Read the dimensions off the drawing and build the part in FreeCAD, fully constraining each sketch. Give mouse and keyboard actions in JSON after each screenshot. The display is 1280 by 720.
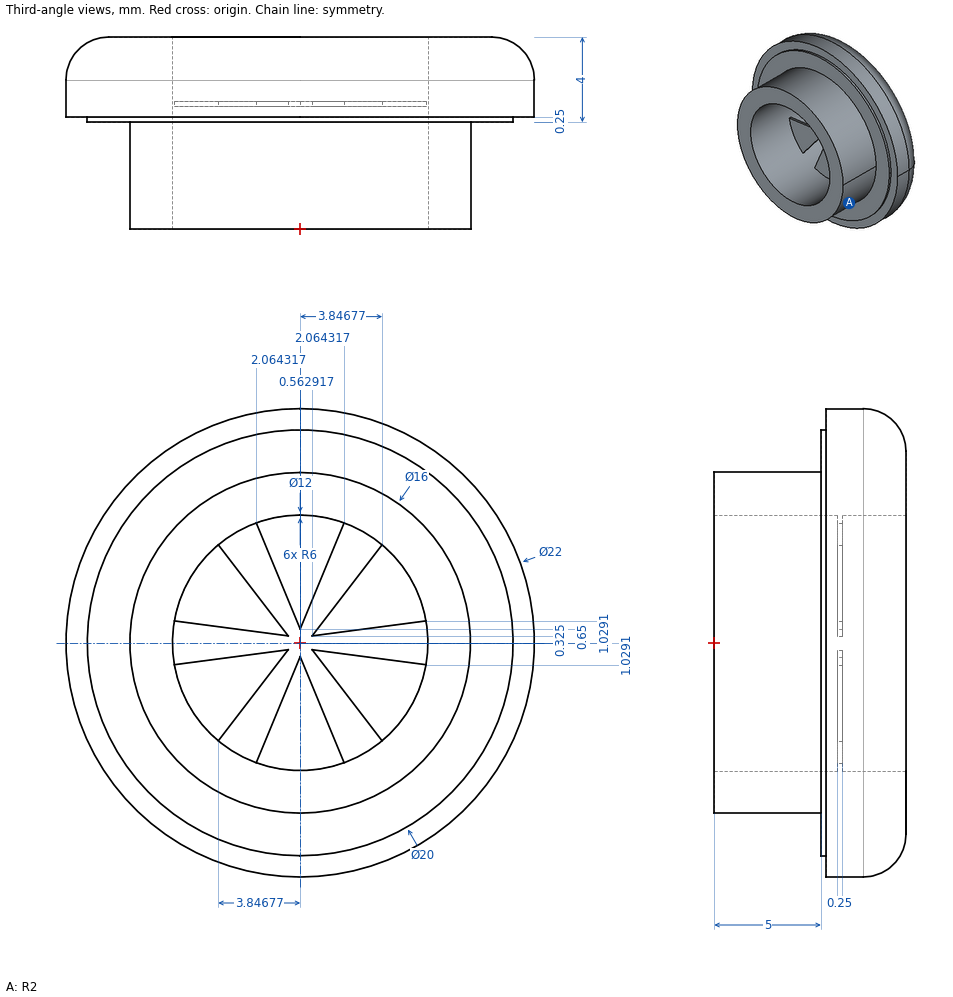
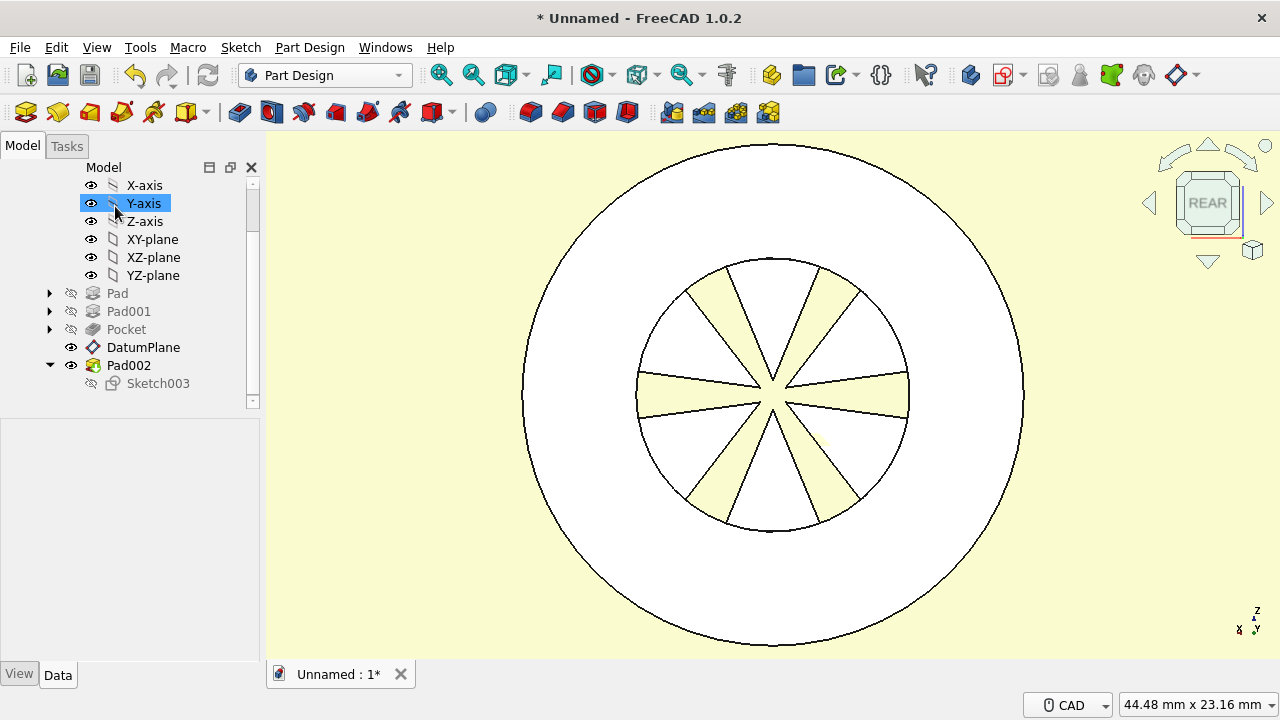
{"action": "left_click", "coordinate": [116, 347]}
{"action": "key", "text": "space"}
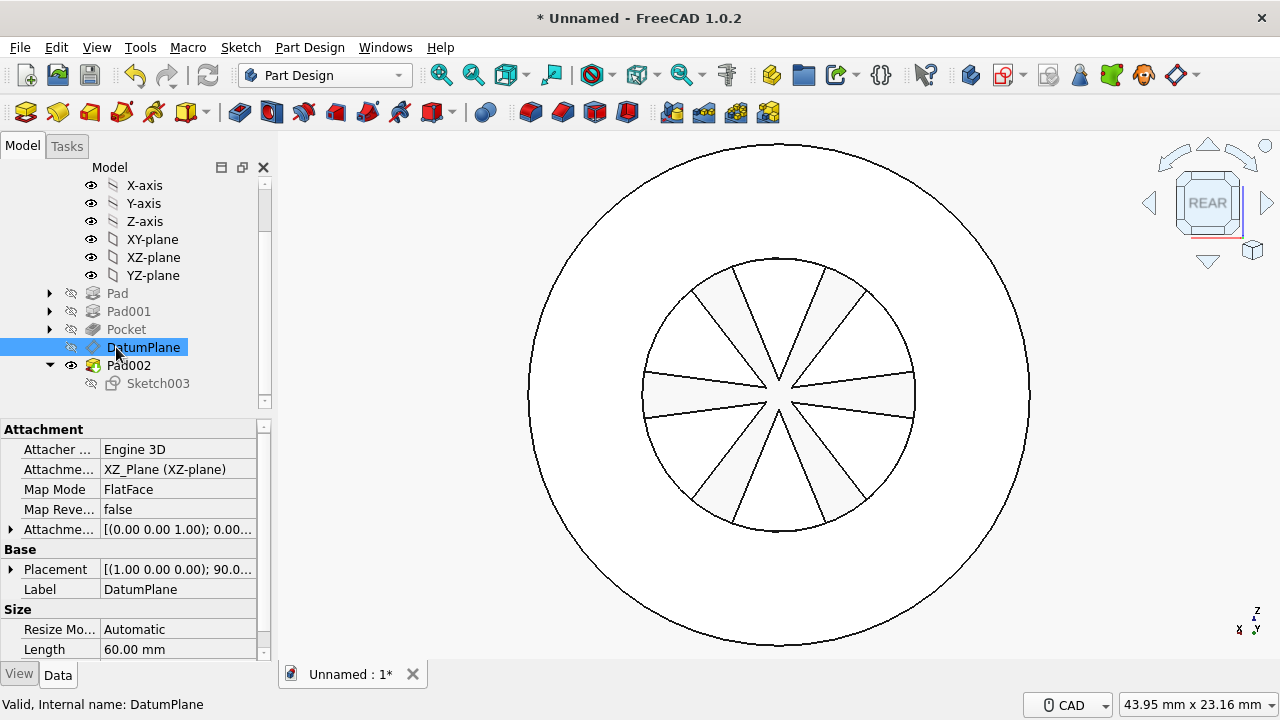
{"action": "key", "text": "0"}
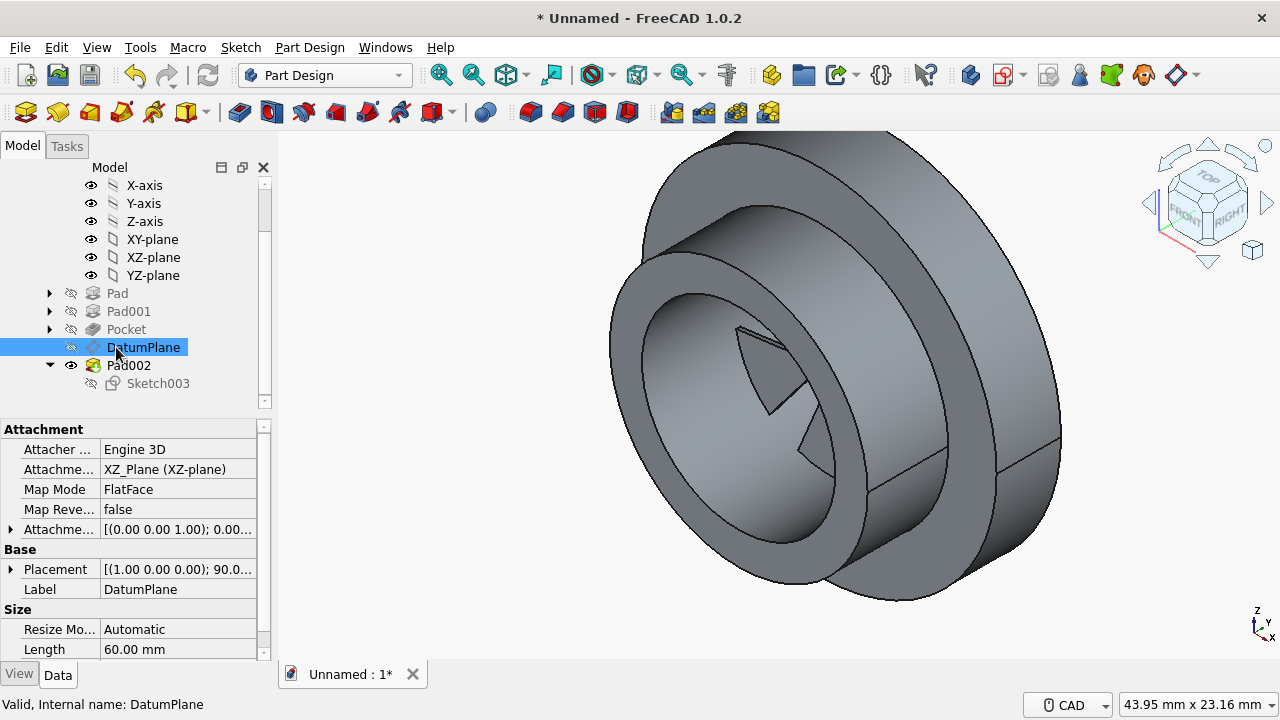
{"action": "key", "text": "v f"}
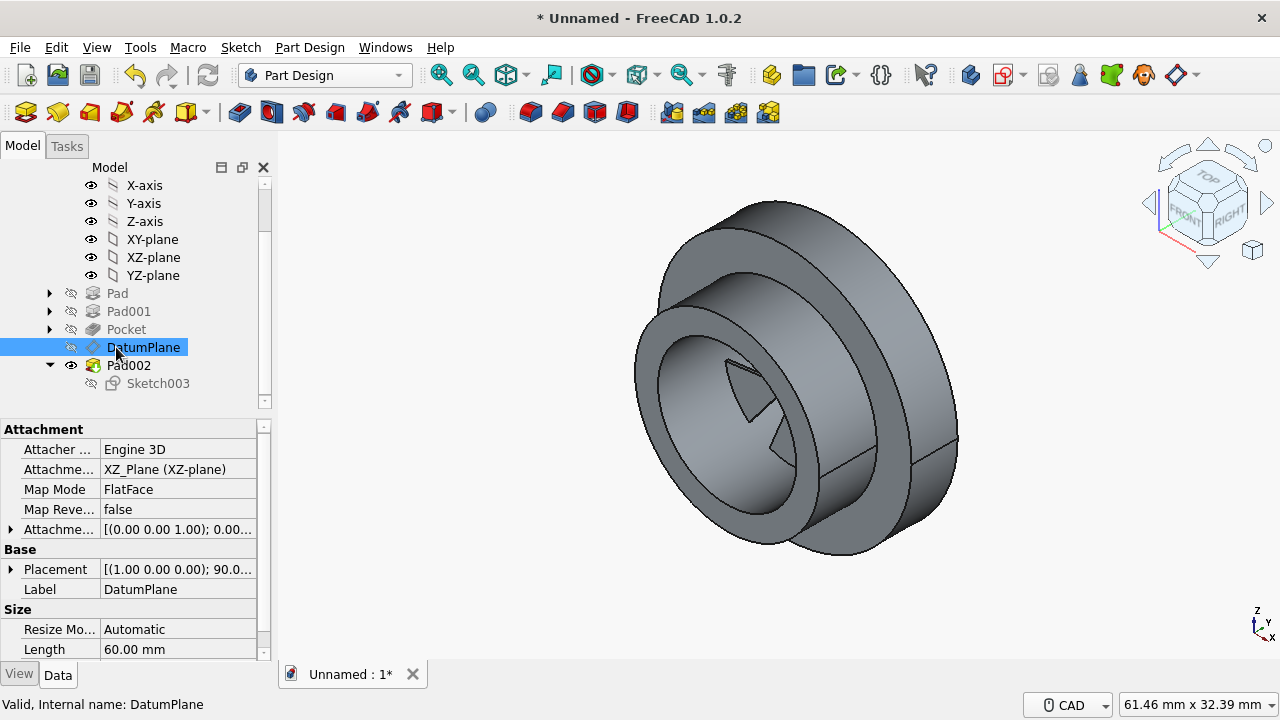
{"action": "left_click", "coordinate": [785, 265]}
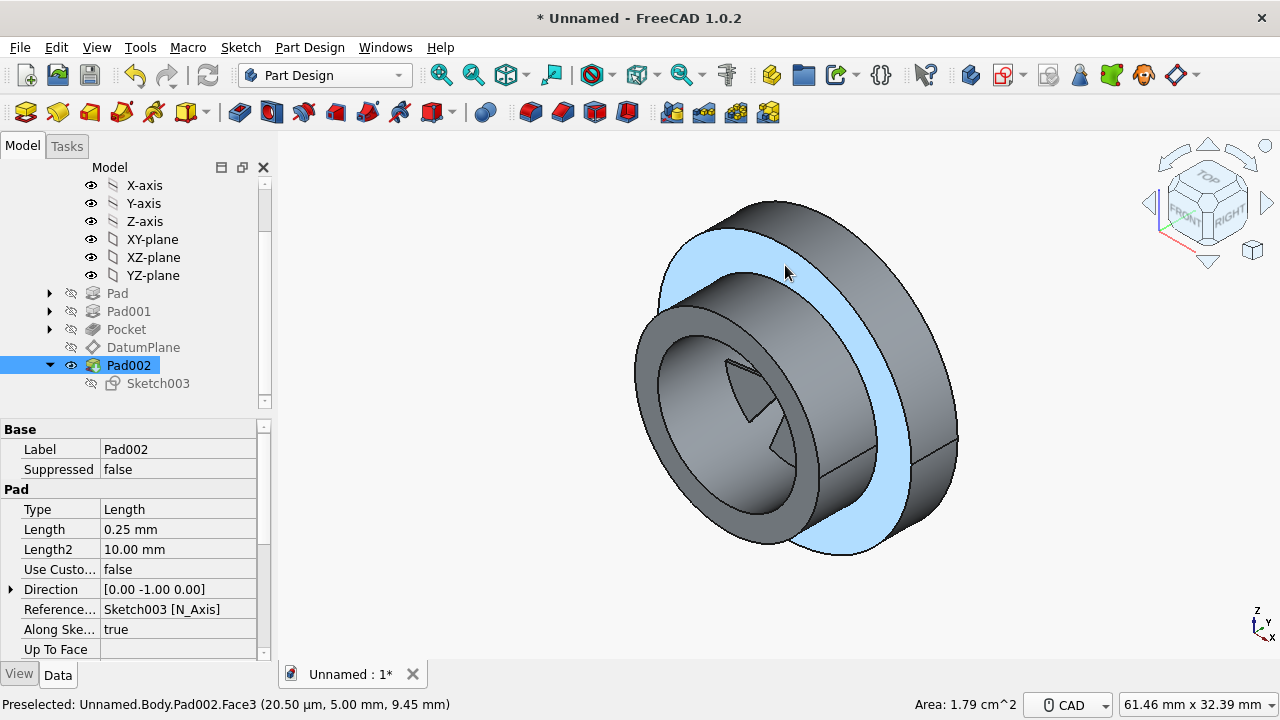
{"action": "left_click", "coordinate": [1004, 76]}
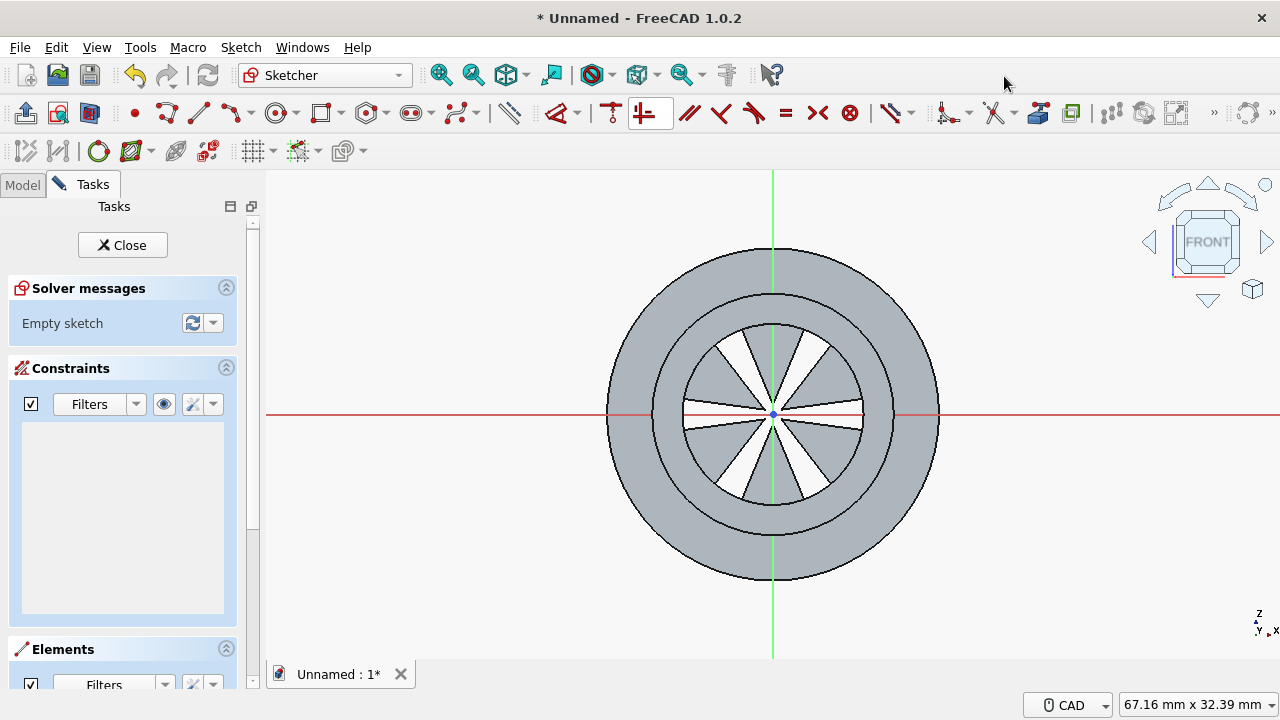
{"action": "key", "text": "g c"}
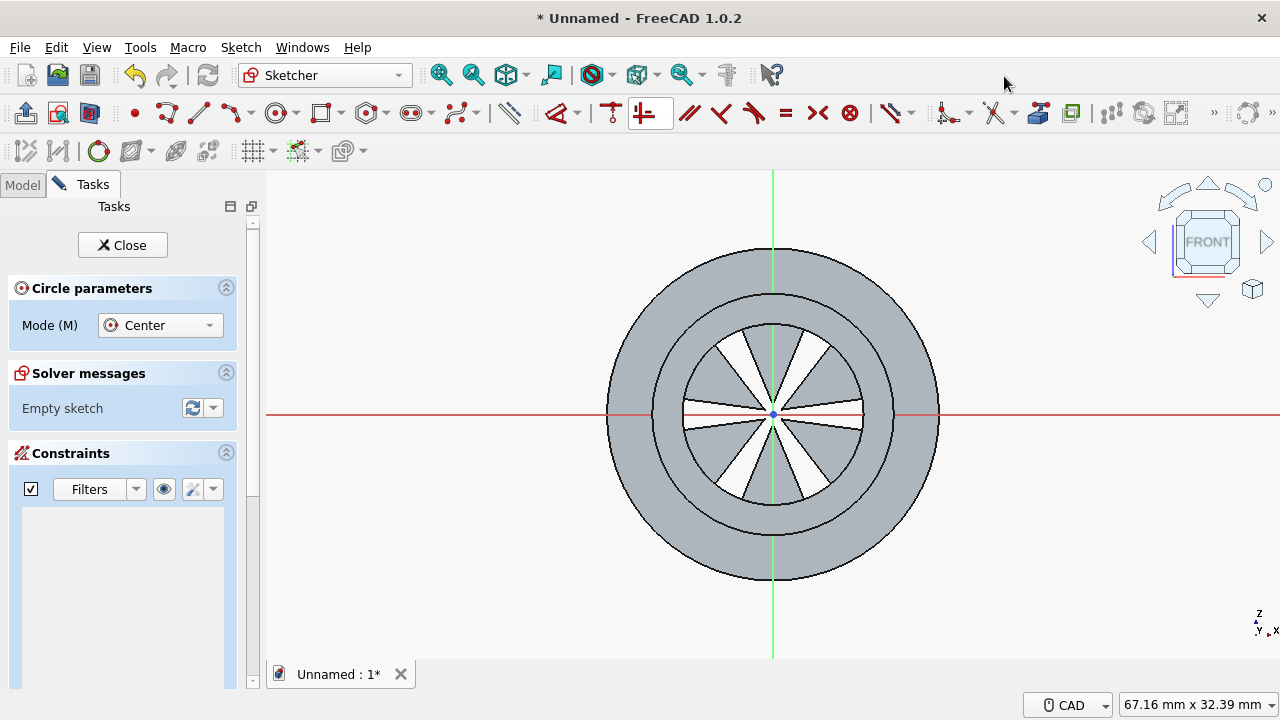
{"action": "left_click", "coordinate": [773, 415]}
{"action": "left_click", "coordinate": [890, 297]}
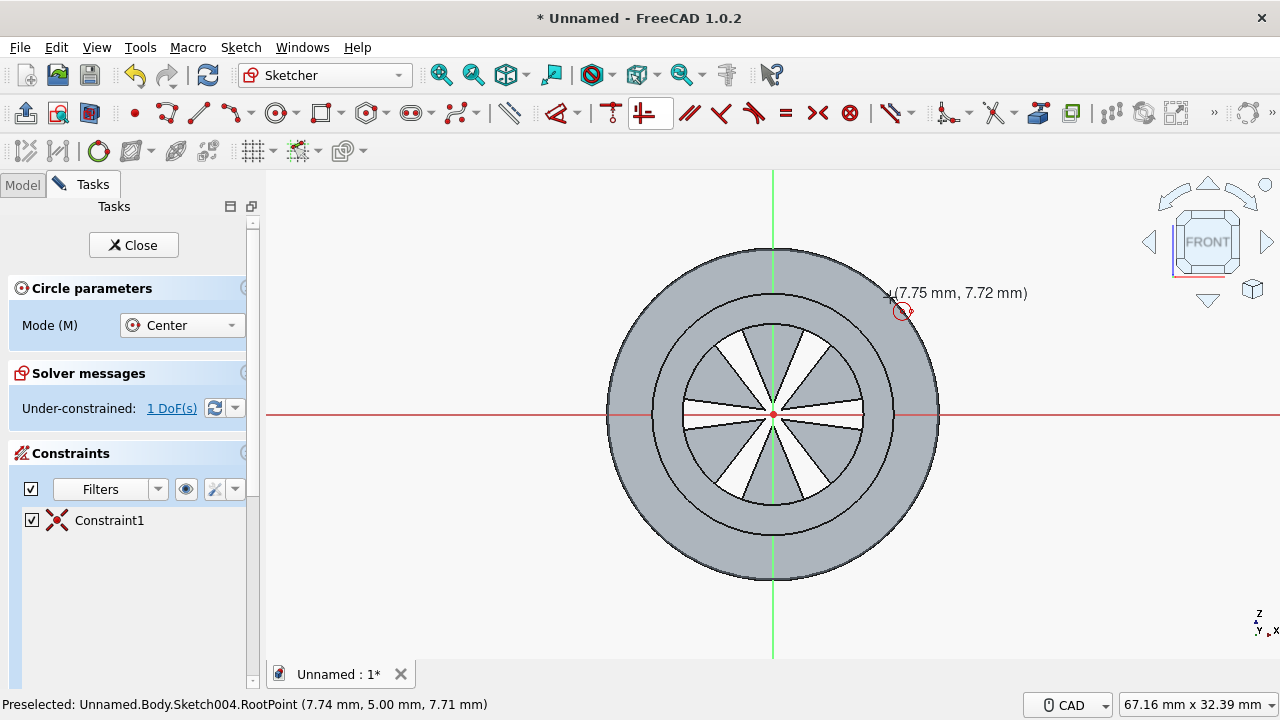
{"action": "left_click", "coordinate": [773, 415]}
{"action": "left_click", "coordinate": [880, 308]}
{"action": "key", "text": "Escape"}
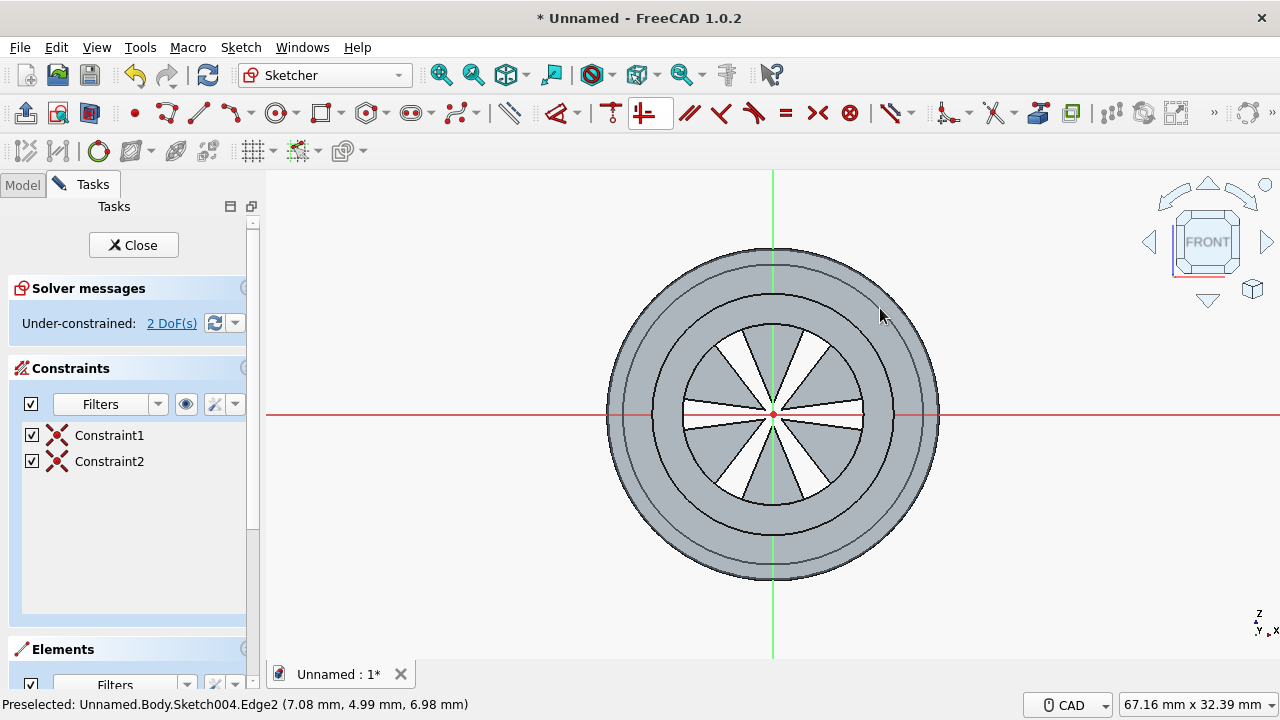
{"action": "key", "text": "d"}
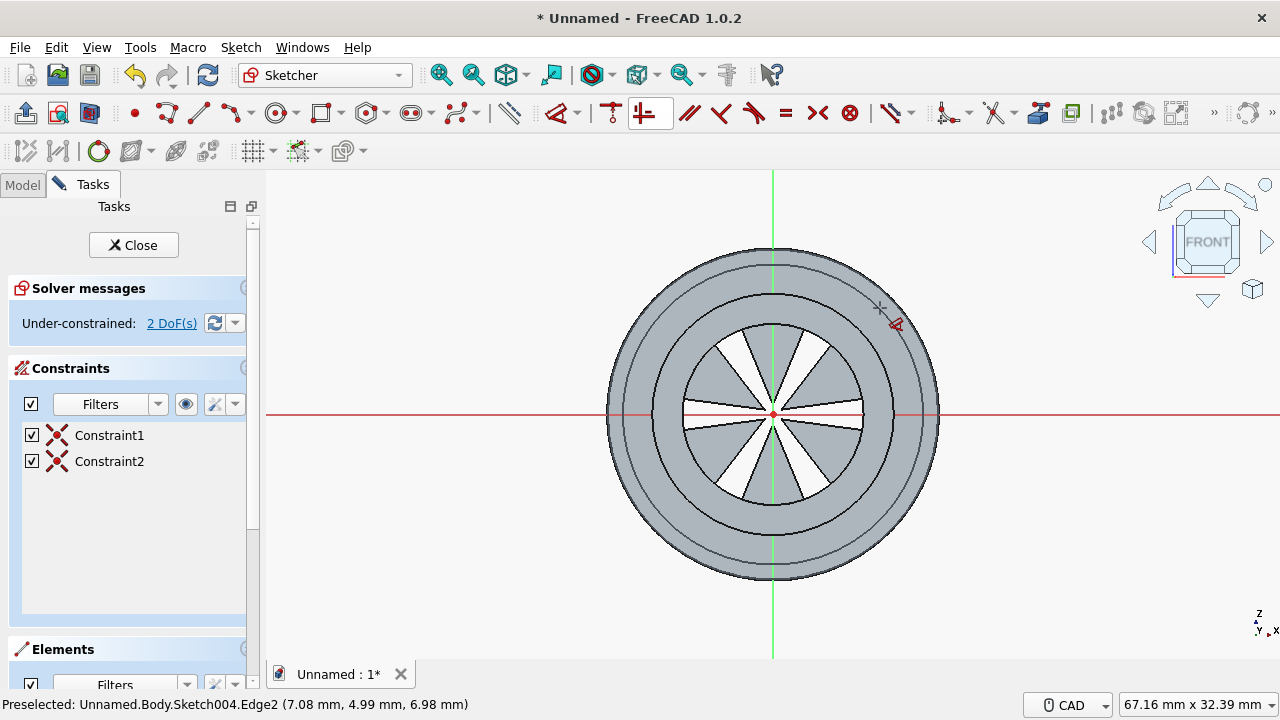
{"action": "left_click", "coordinate": [889, 297]}
{"action": "left_click", "coordinate": [911, 274]}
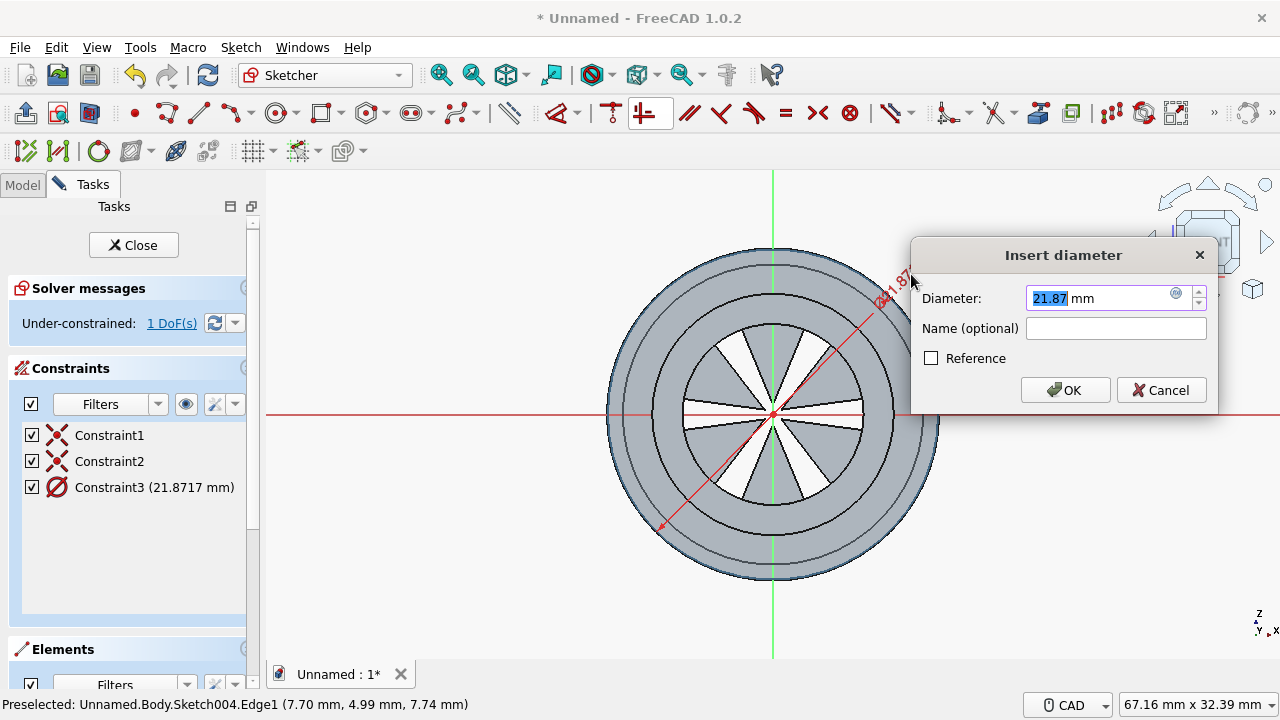
{"action": "type", "text": "22"}
{"action": "key", "text": "Return"}